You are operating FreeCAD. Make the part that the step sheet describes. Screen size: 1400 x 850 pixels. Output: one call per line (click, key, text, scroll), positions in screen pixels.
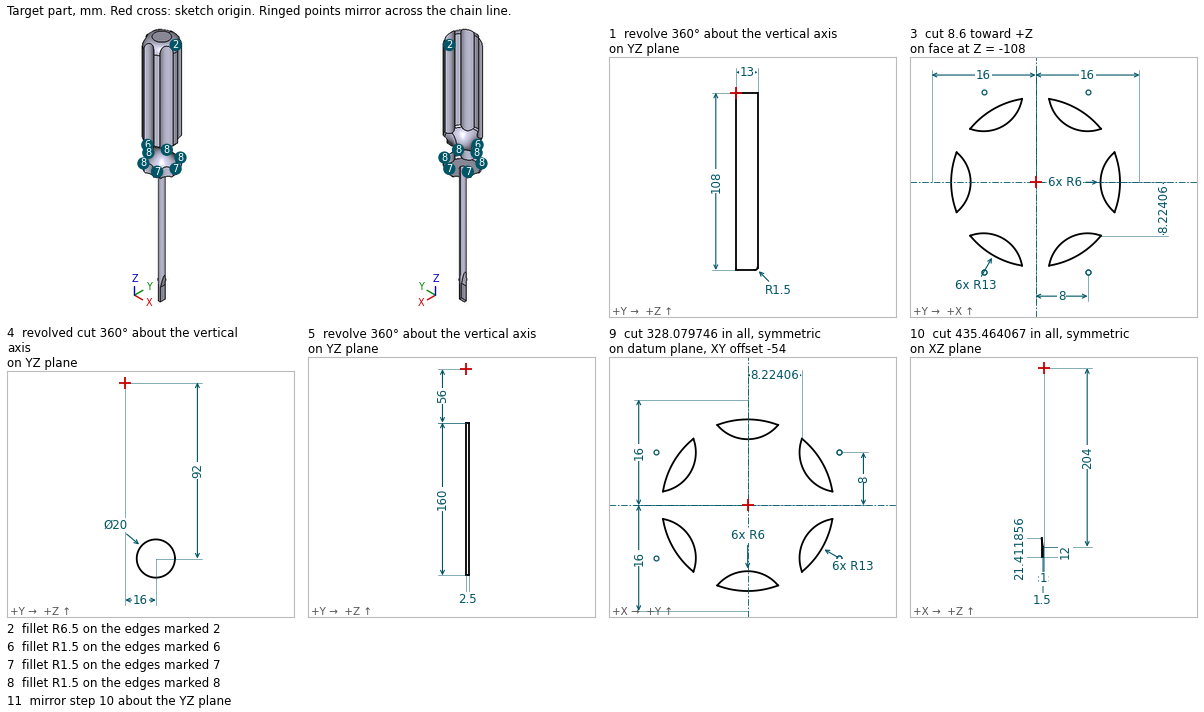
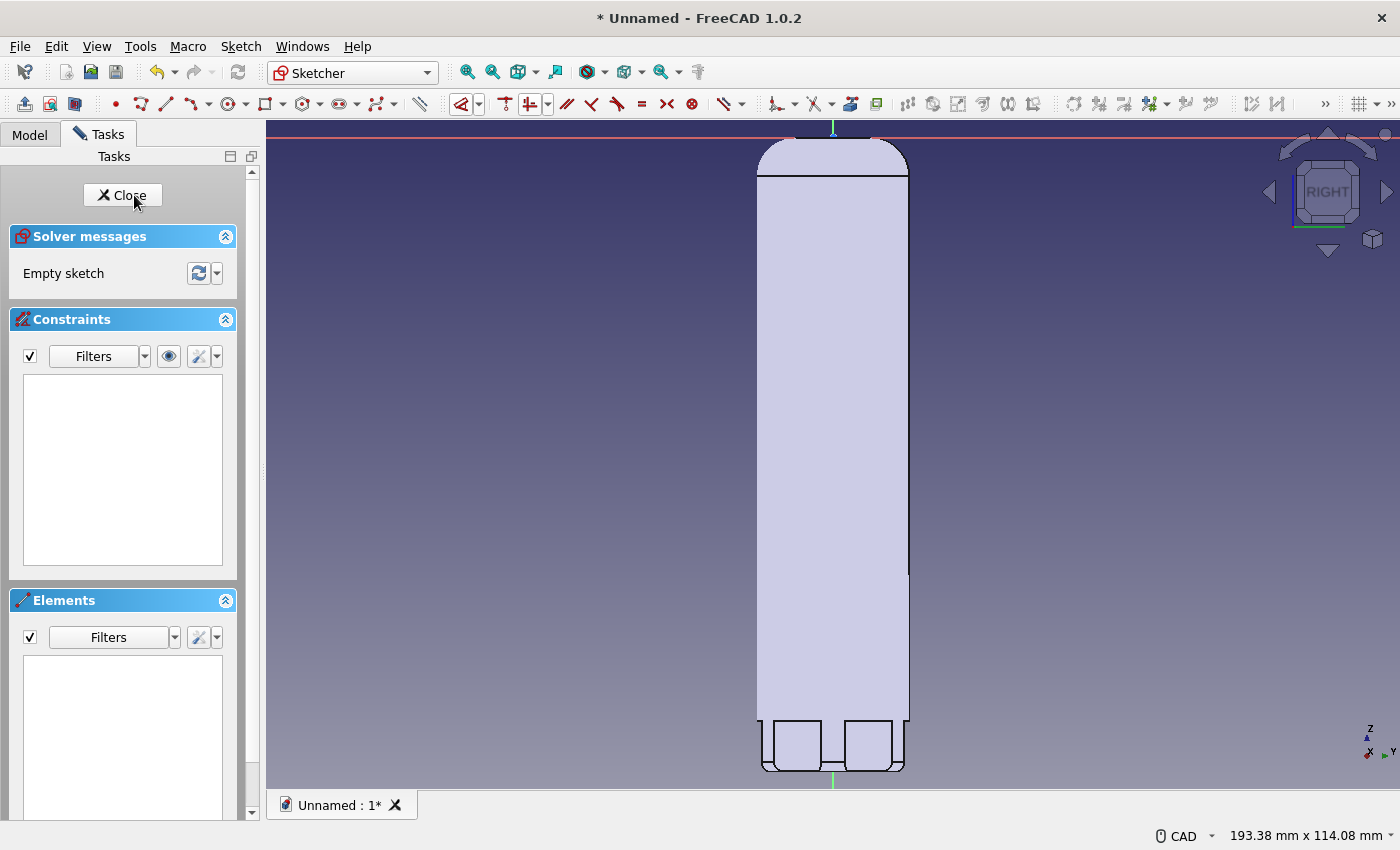
key(q)
key(s)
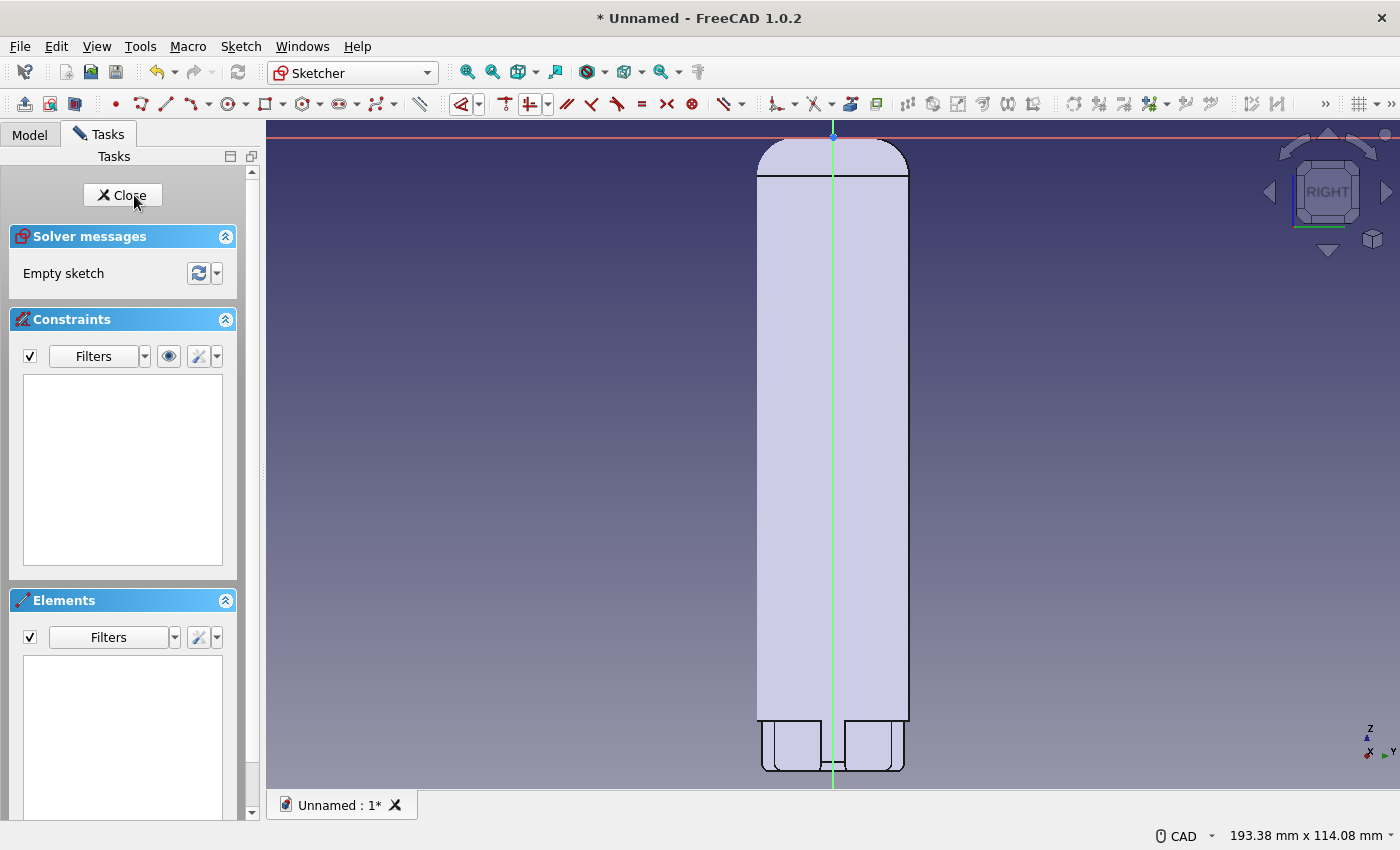
scroll(980, 750, up, 7)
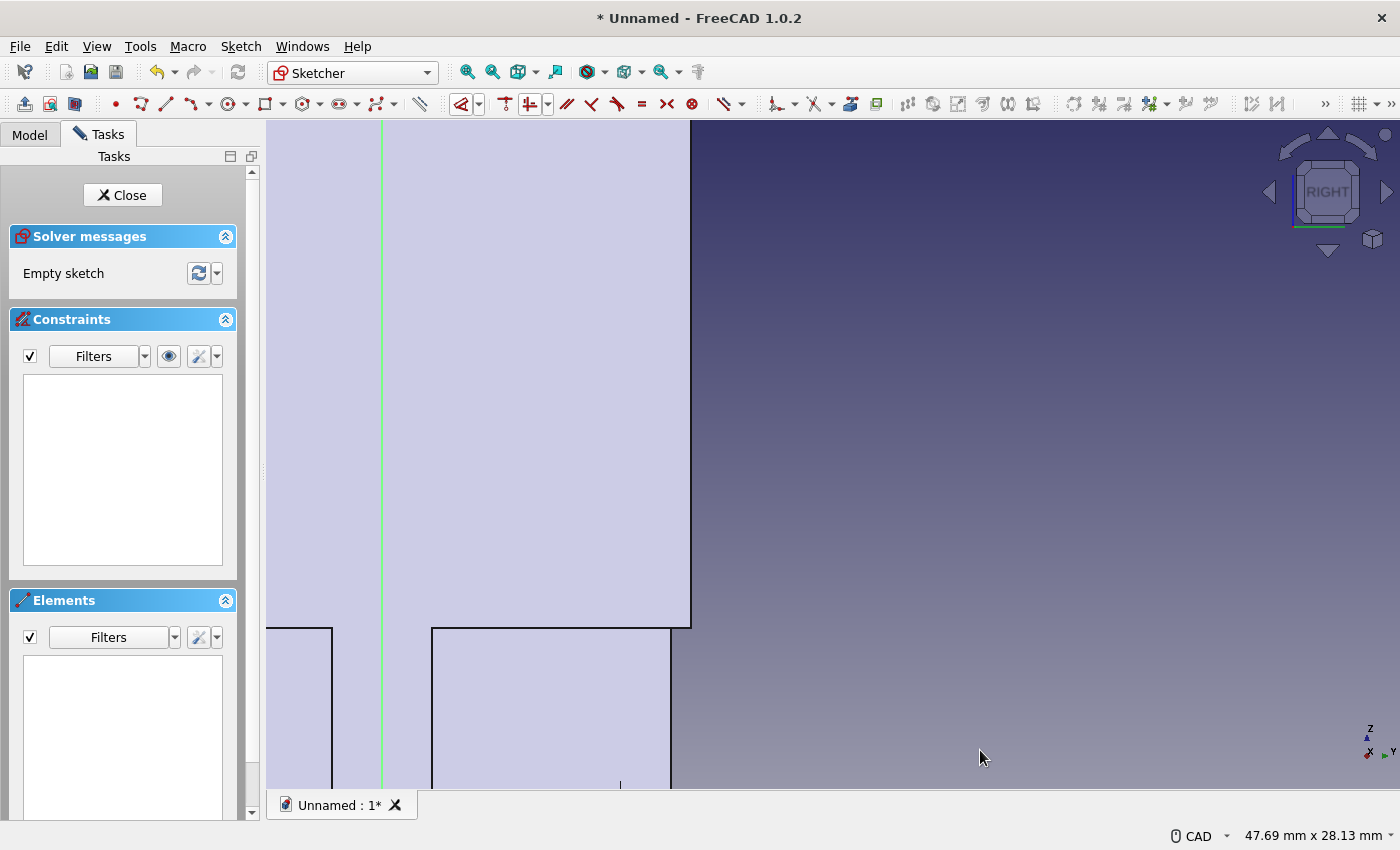
key(g)
key(c)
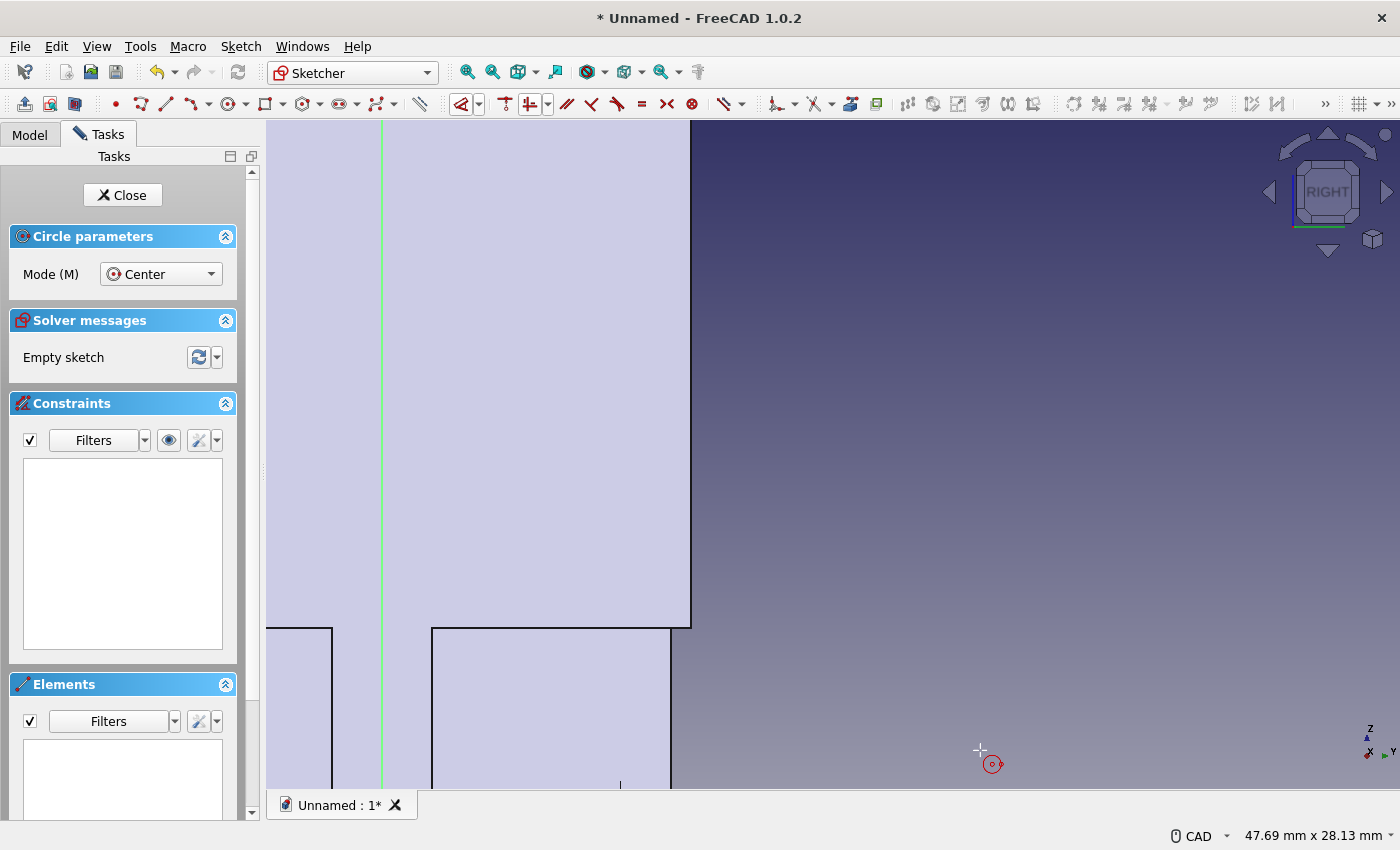
click(762, 452)
move(931, 284)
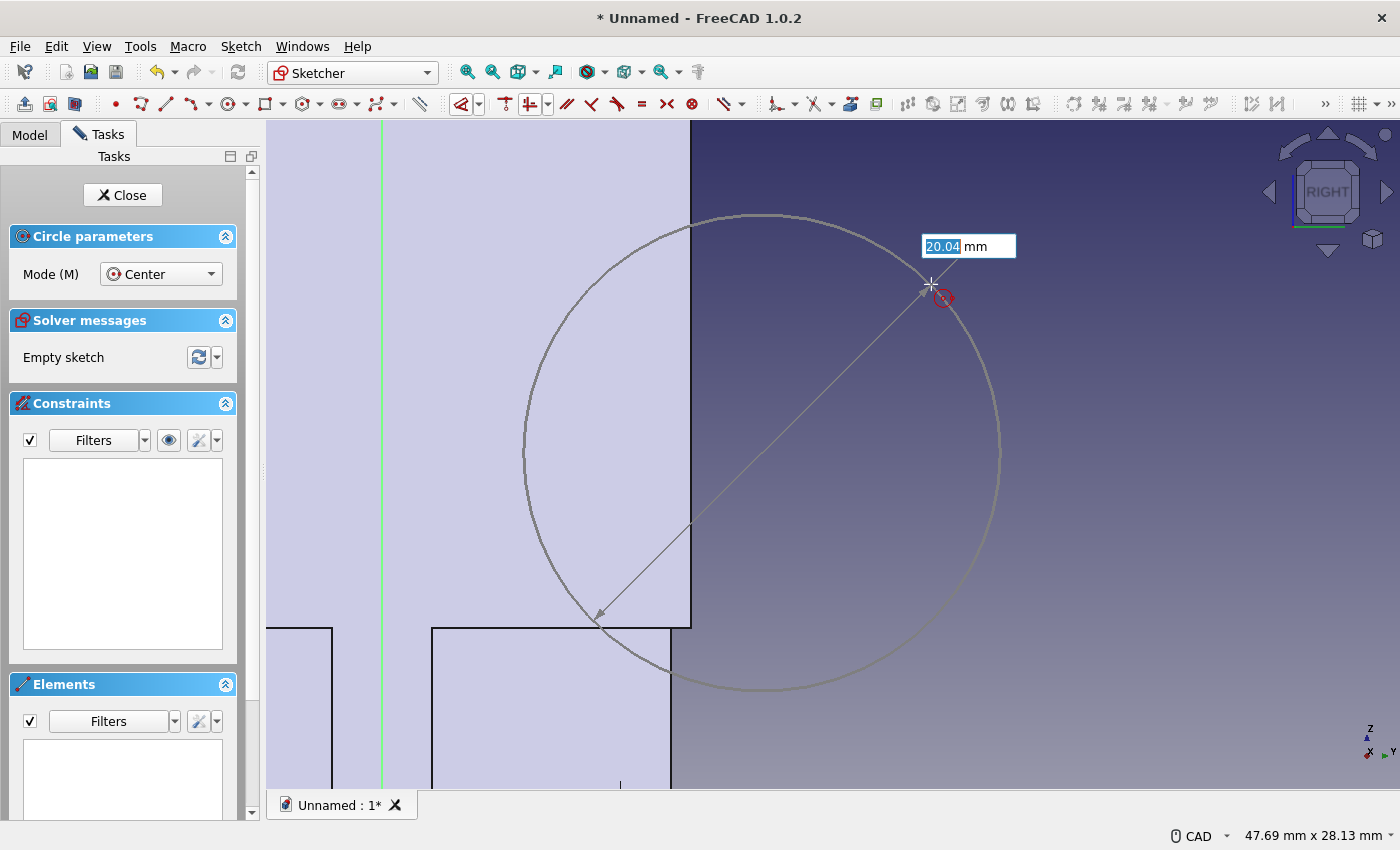
text(20)
key(Return)
key(Escape)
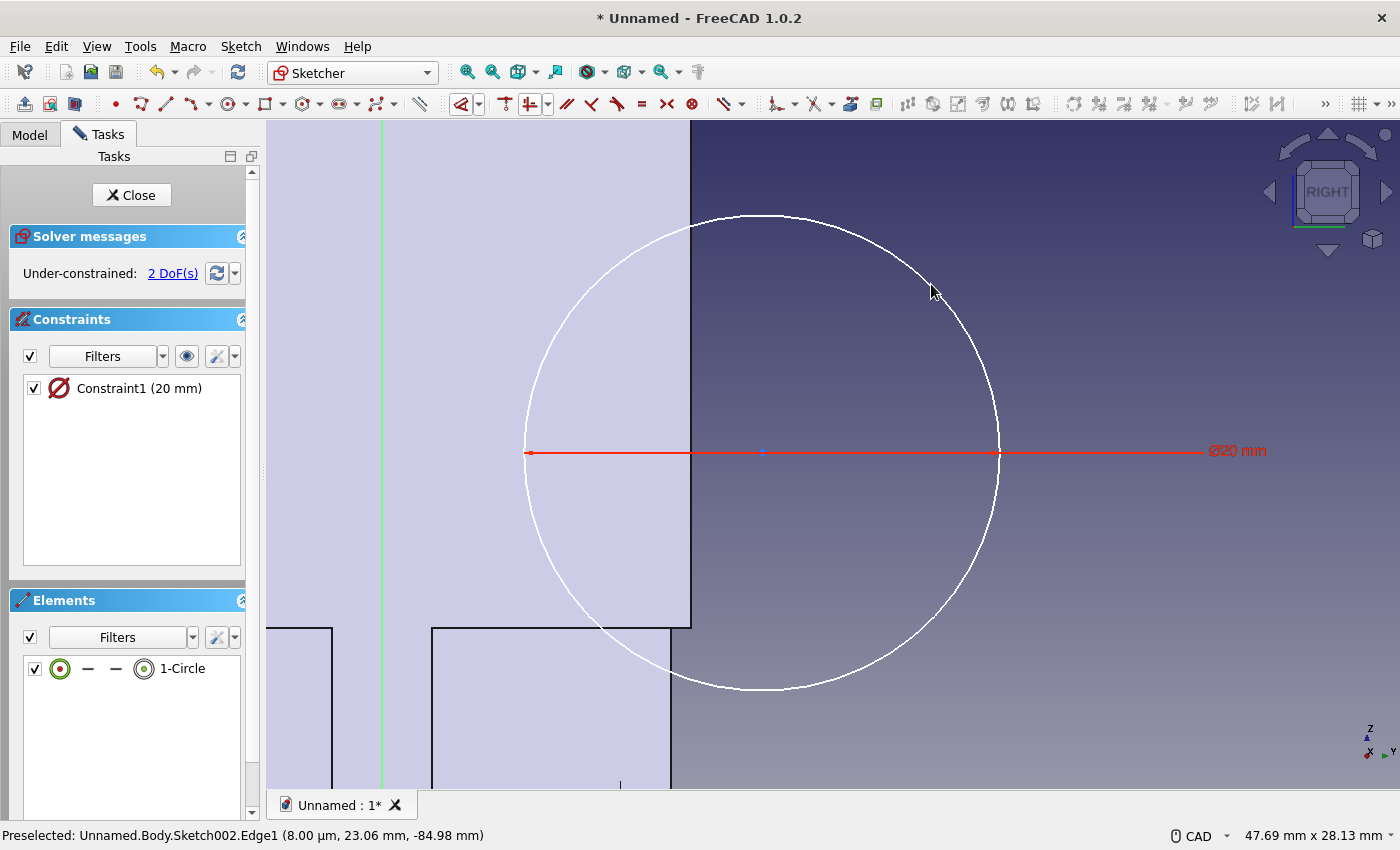
key(d)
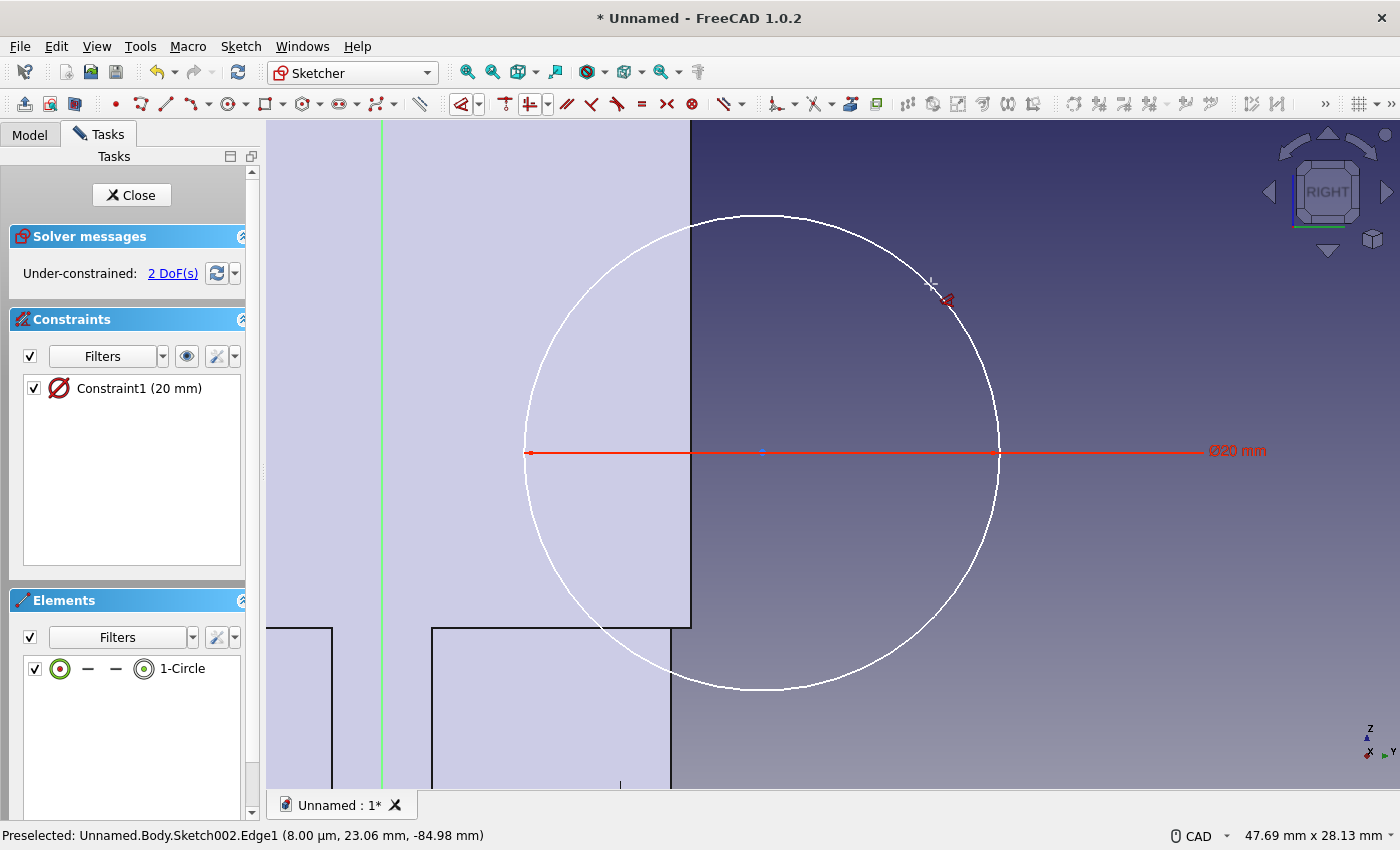
click(762, 453)
click(572, 487)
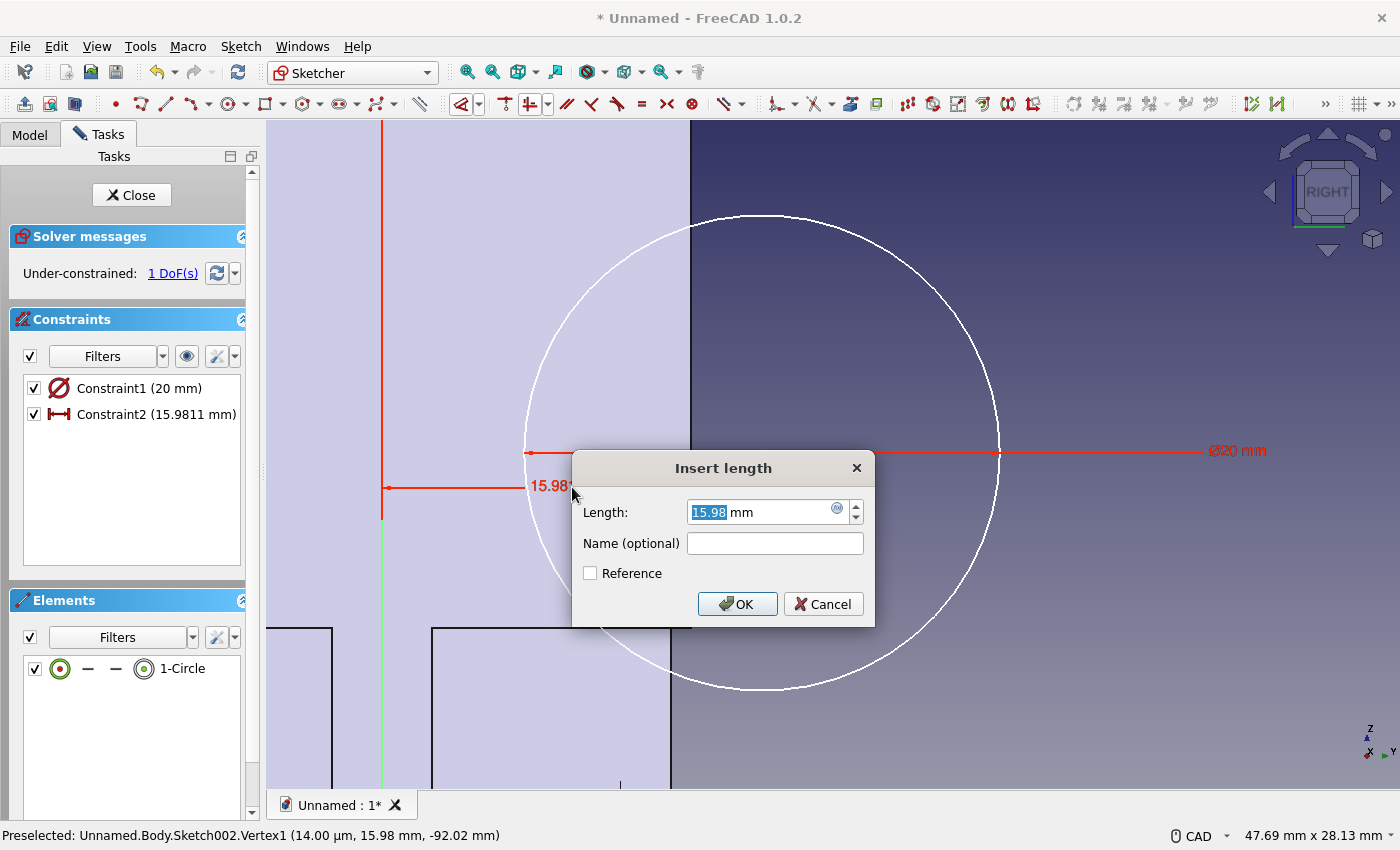
text(16)
key(Return)